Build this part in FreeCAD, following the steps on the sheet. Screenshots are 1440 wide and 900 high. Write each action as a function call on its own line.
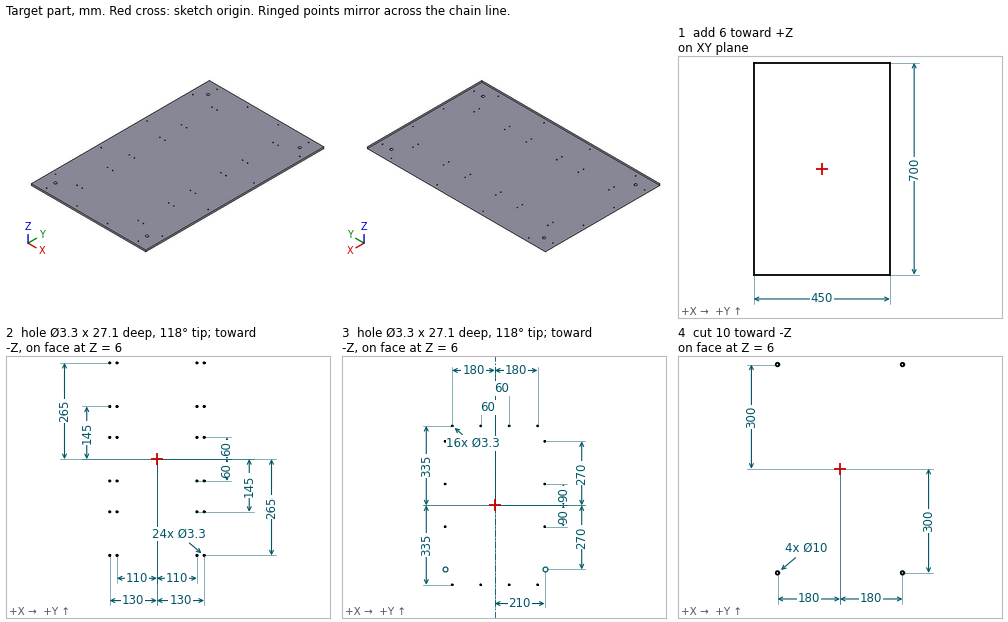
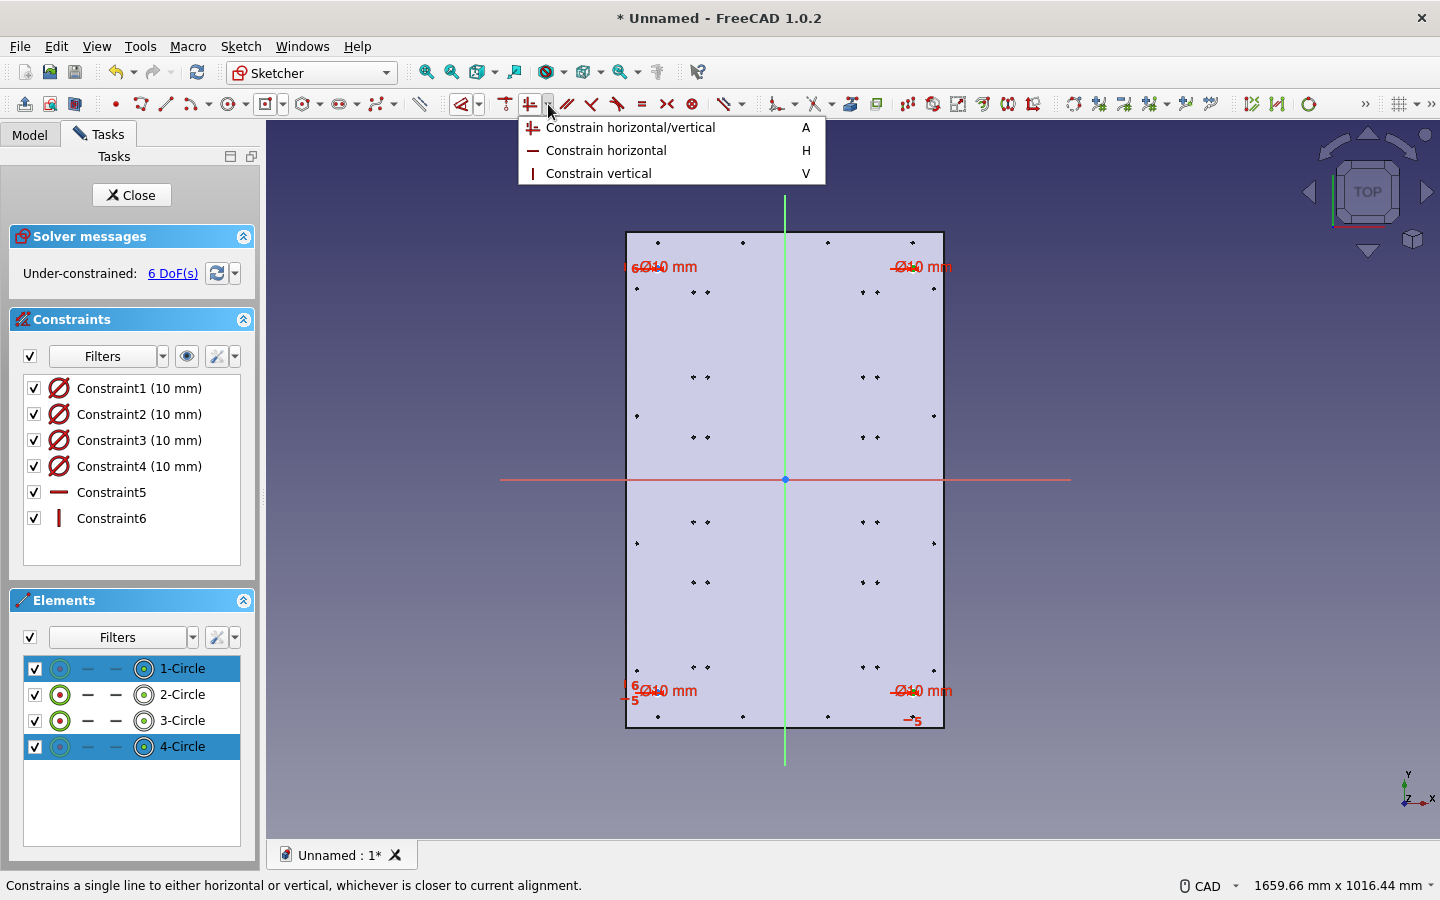
click(672, 174)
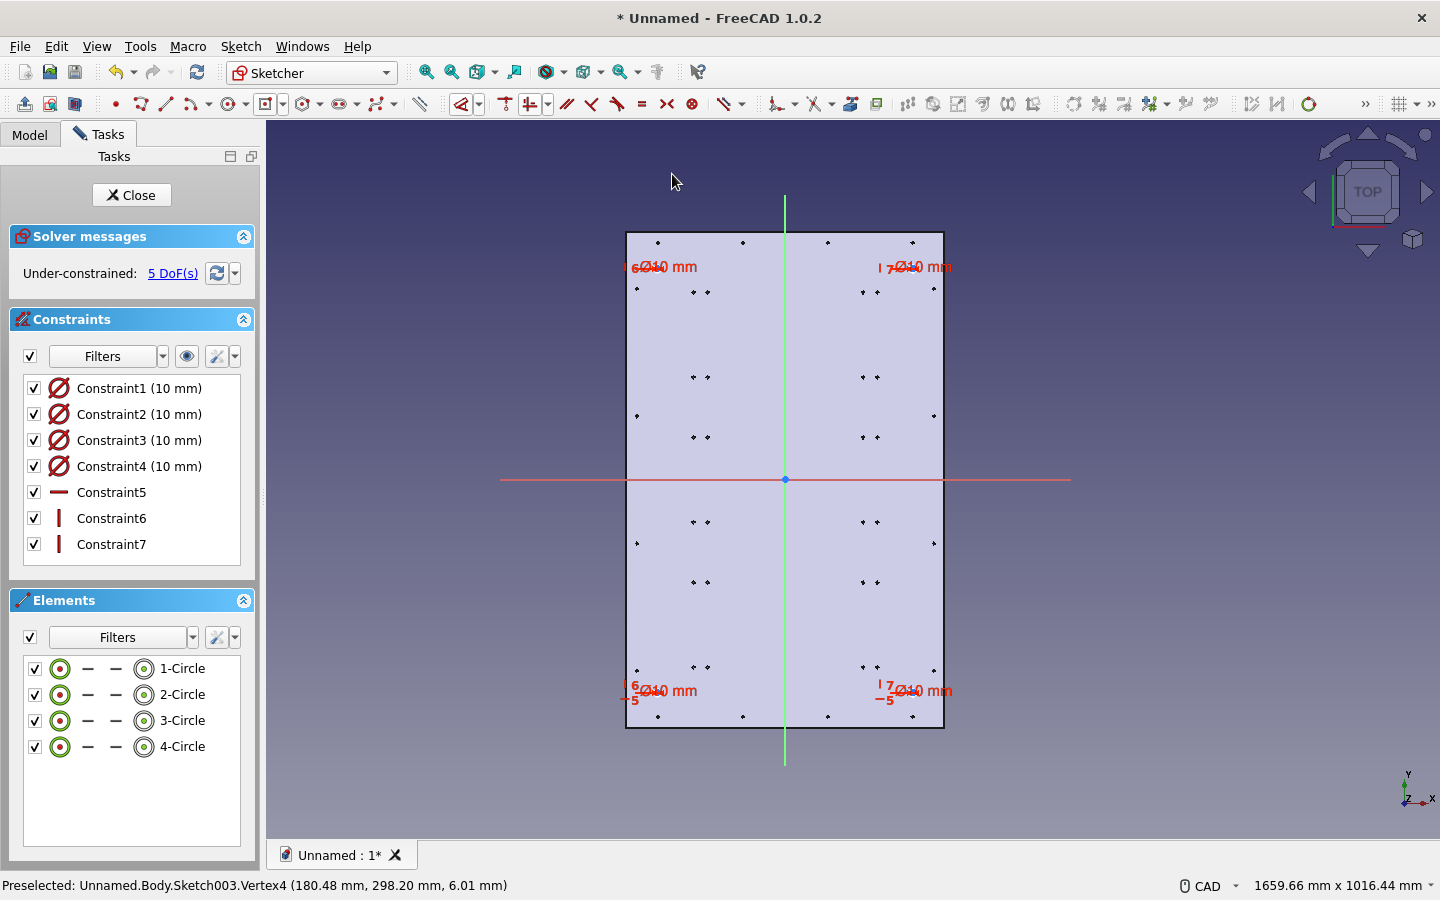
click(658, 269)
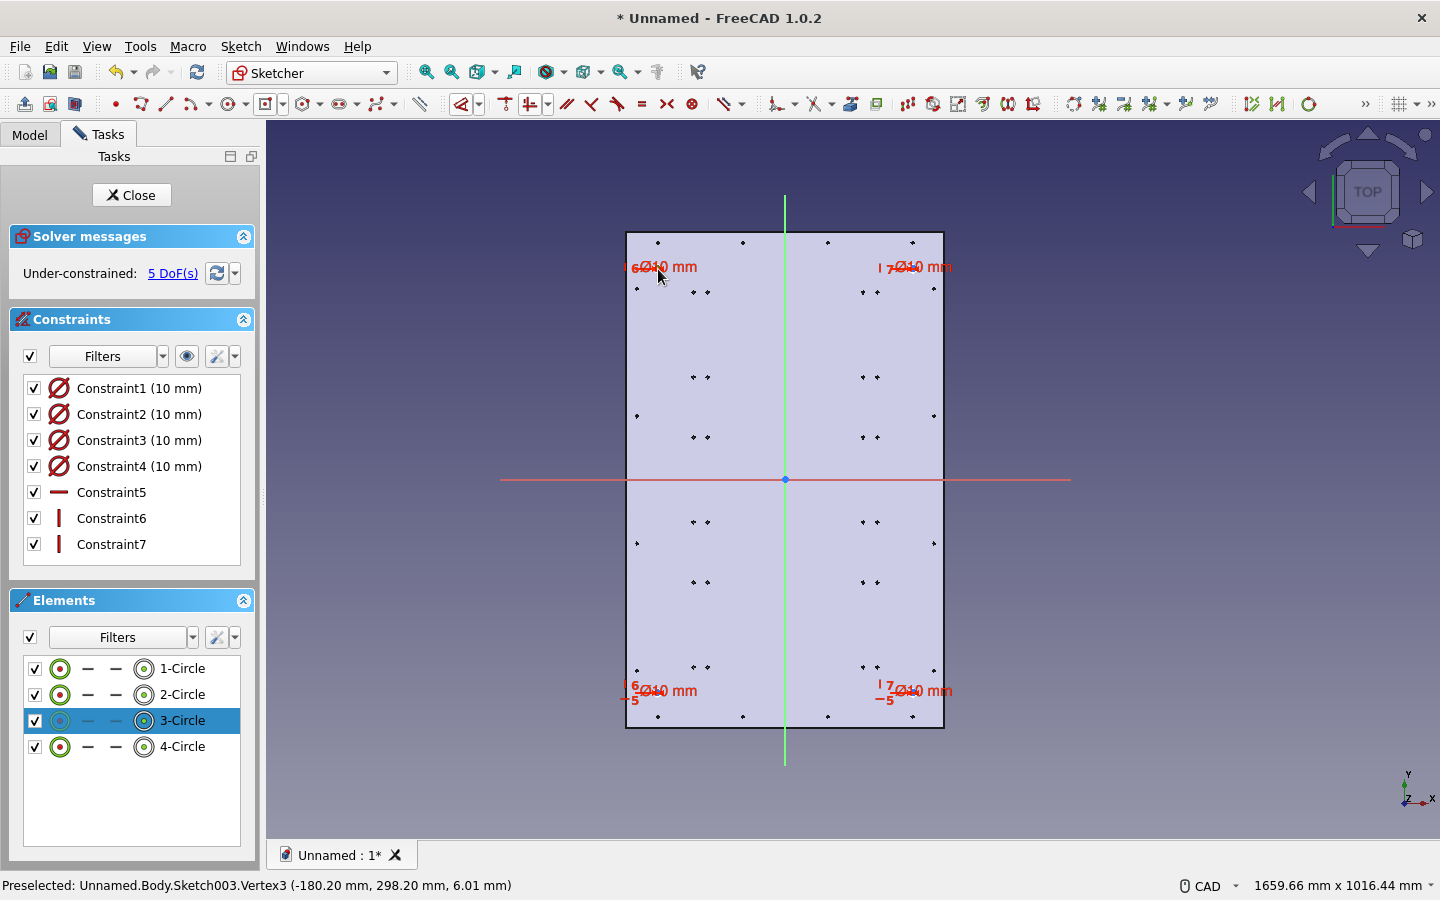
click(913, 269)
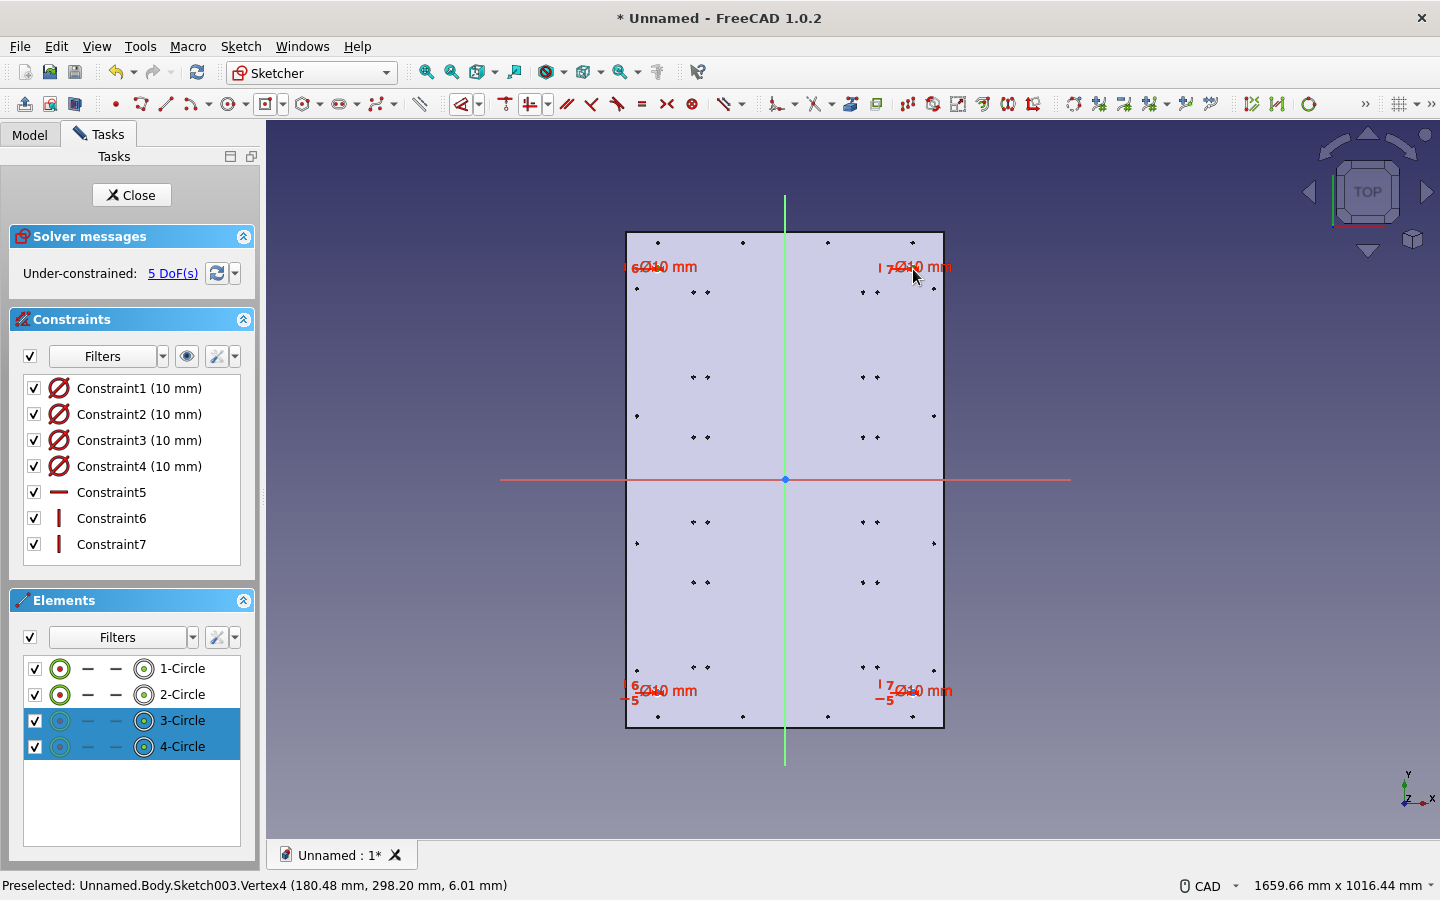
click(548, 104)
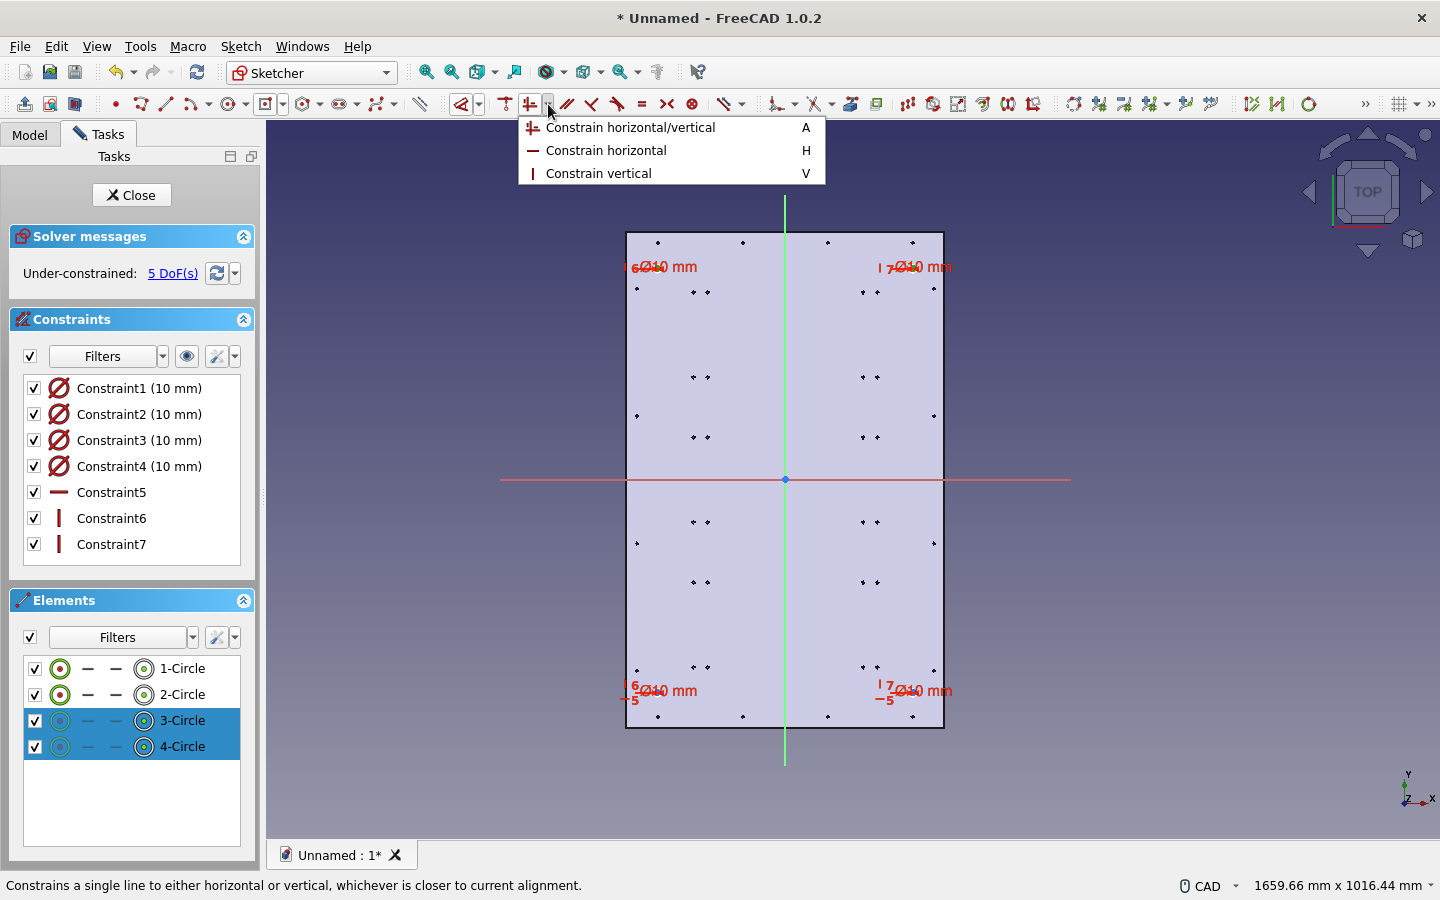
click(672, 150)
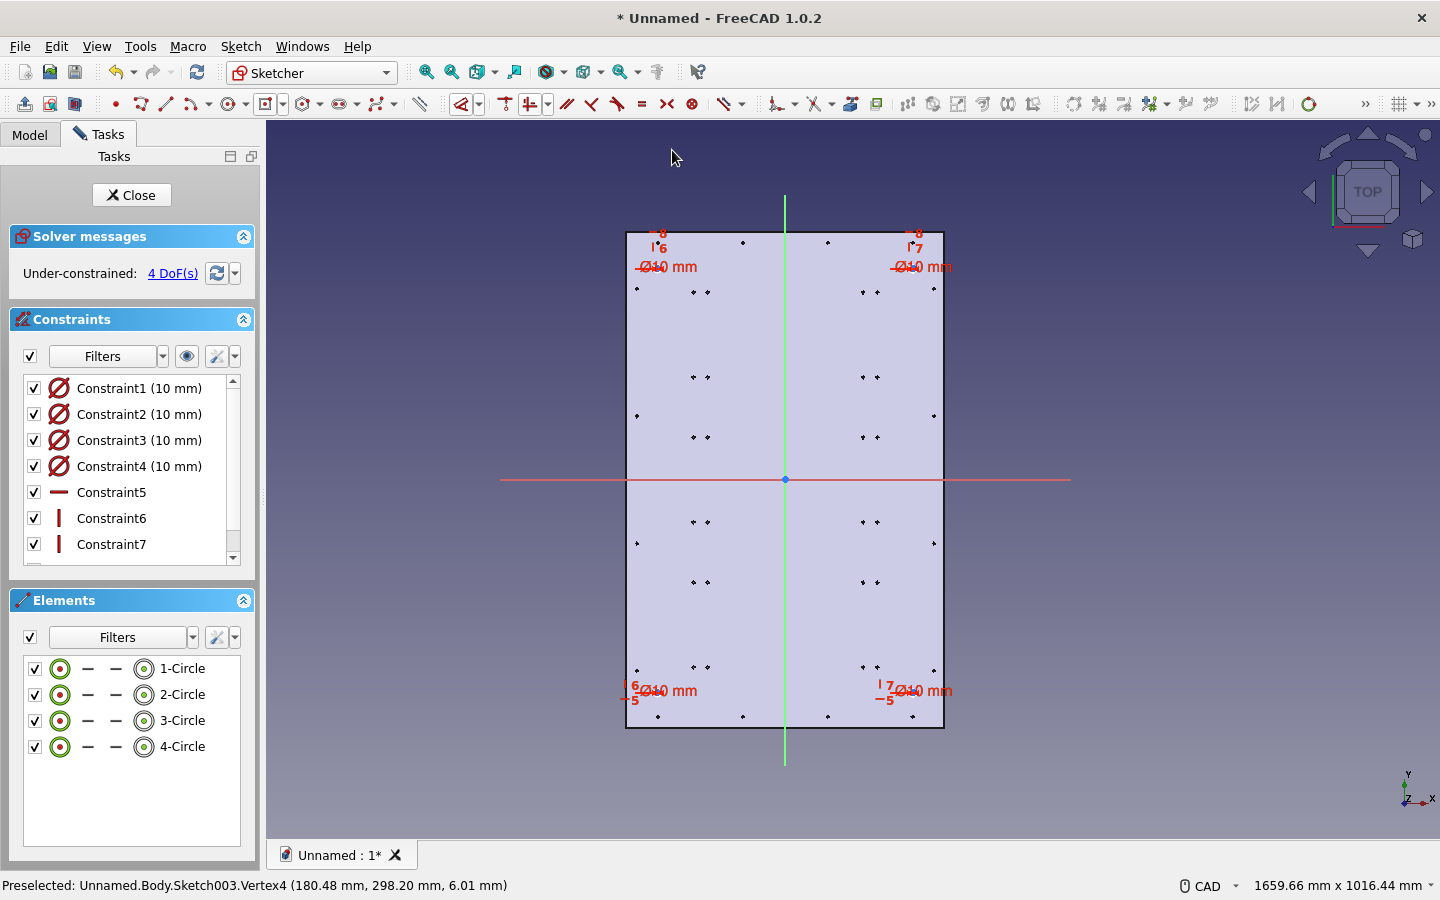
click(913, 693)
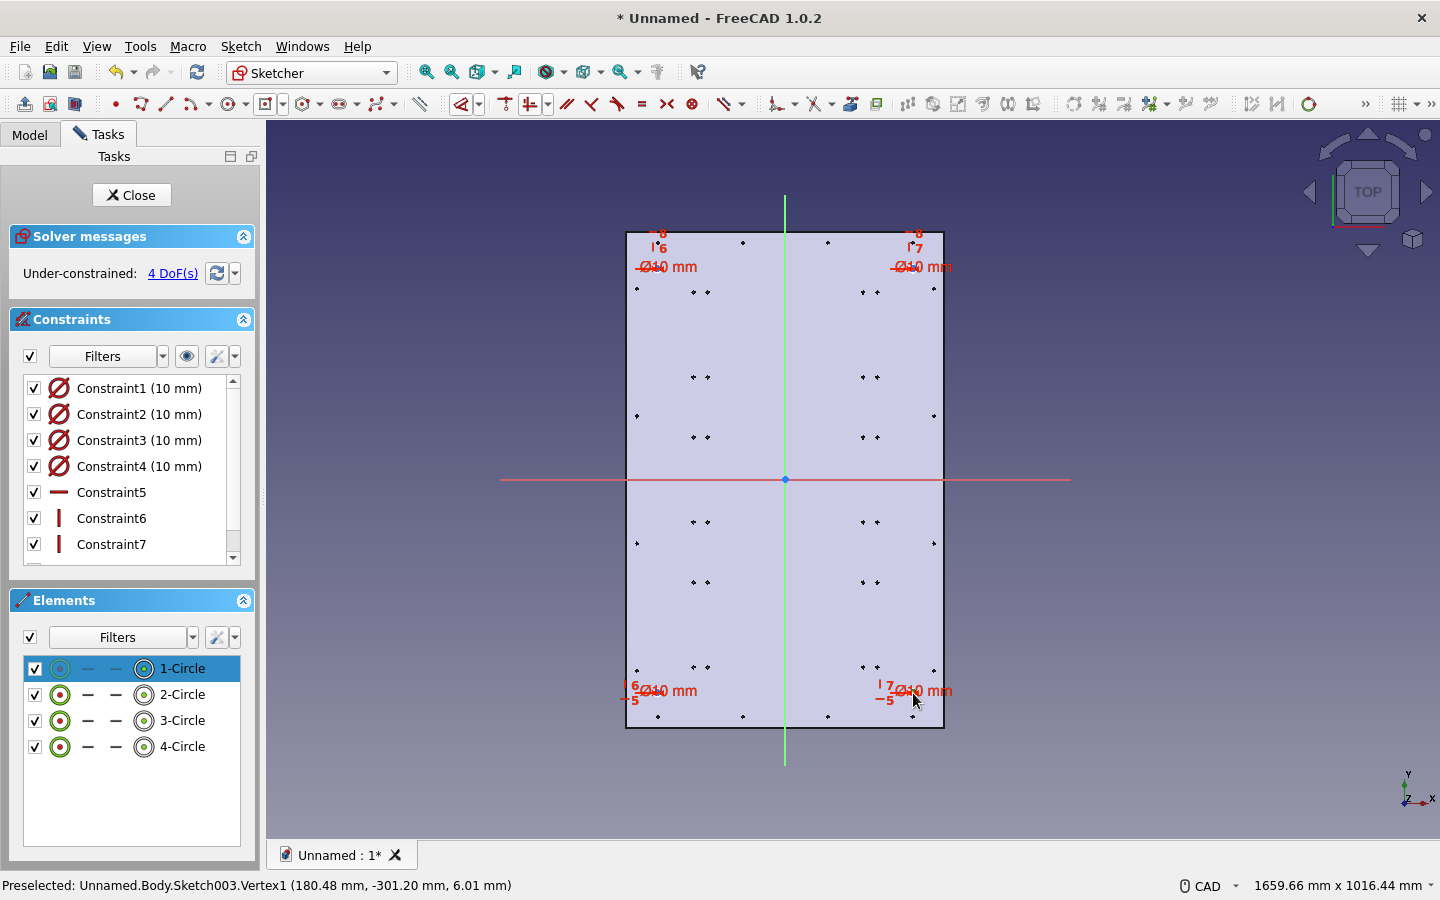
click(478, 104)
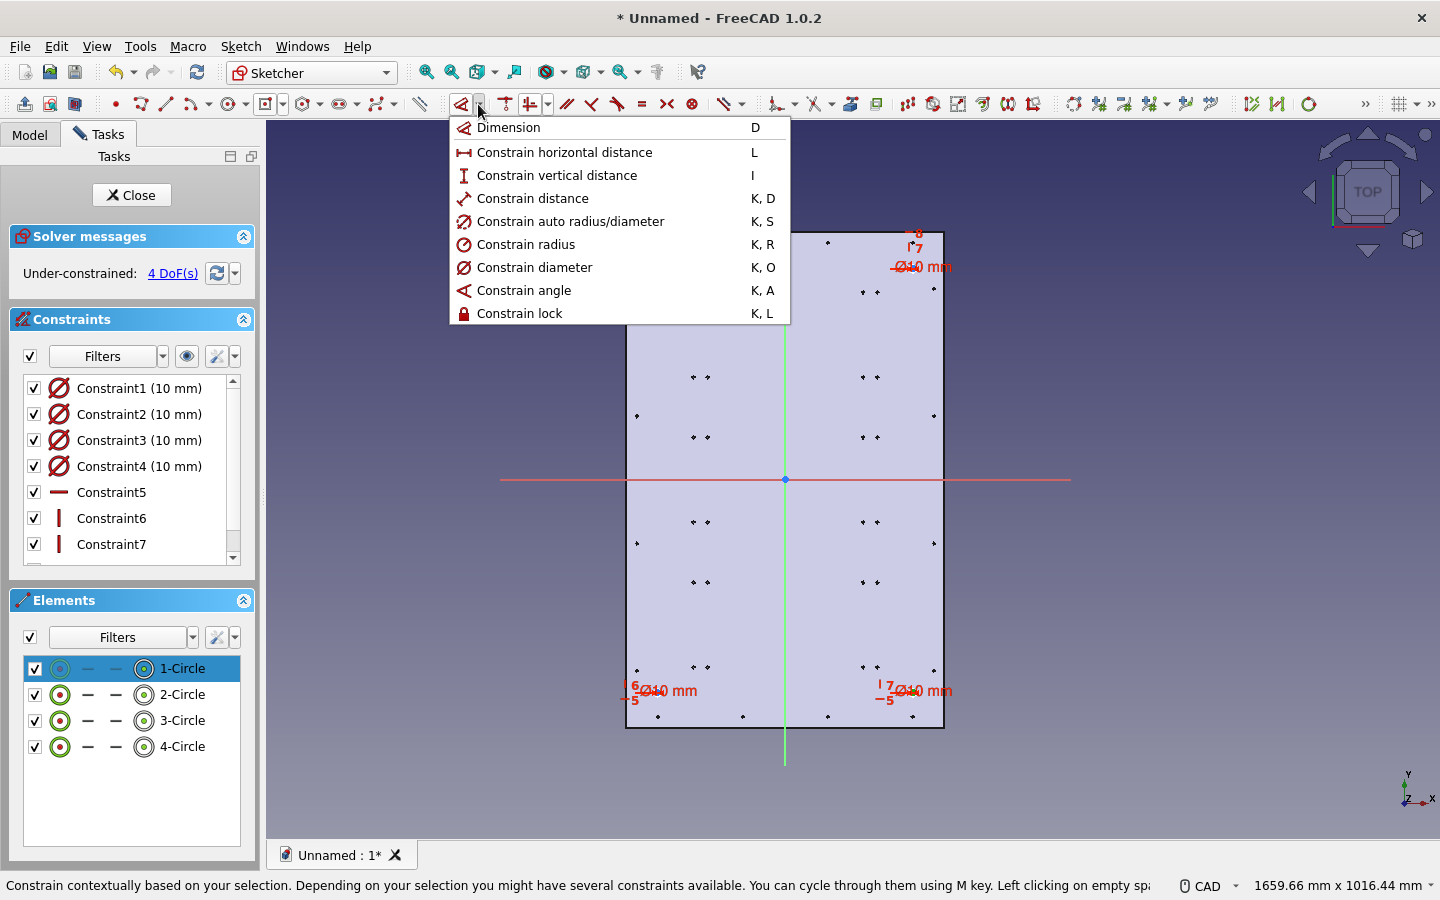
click(620, 152)